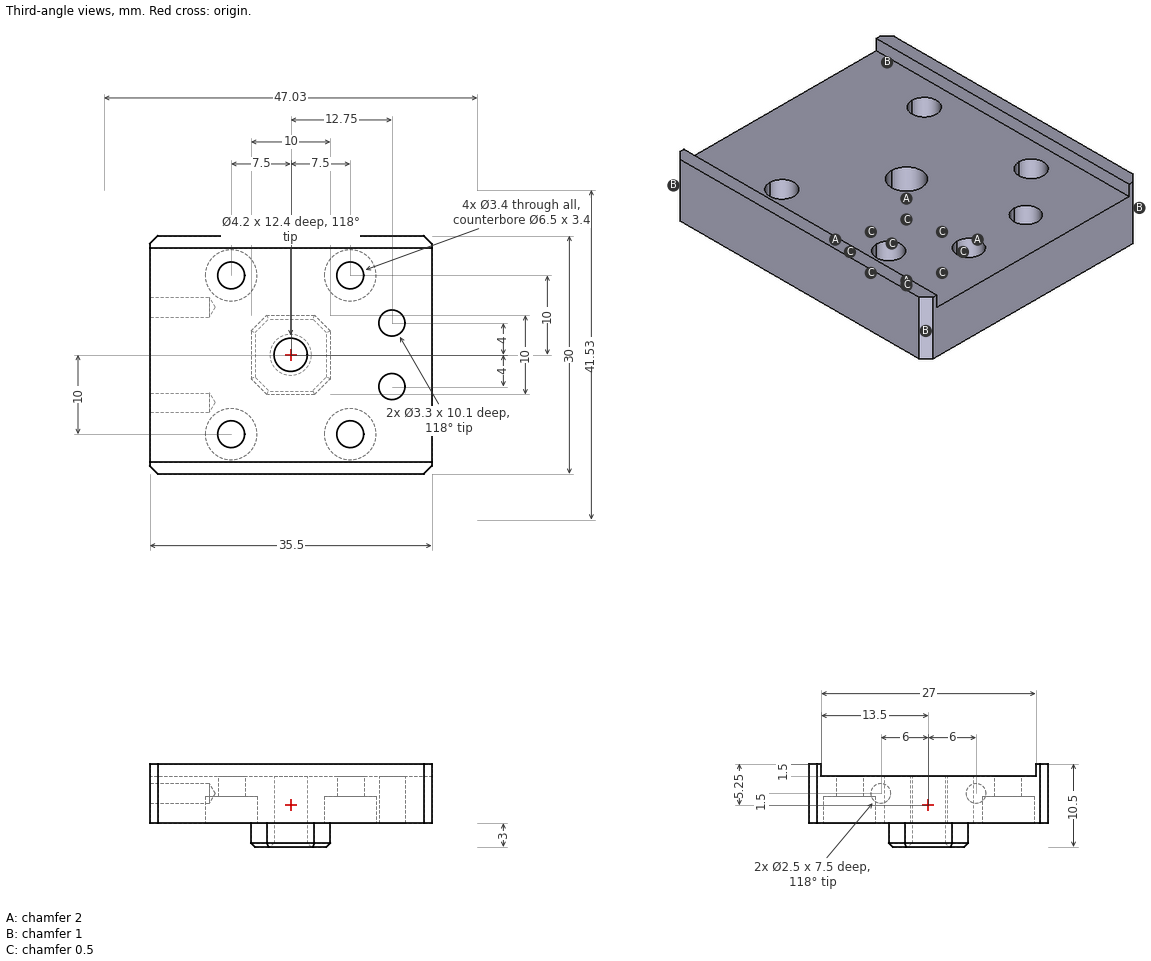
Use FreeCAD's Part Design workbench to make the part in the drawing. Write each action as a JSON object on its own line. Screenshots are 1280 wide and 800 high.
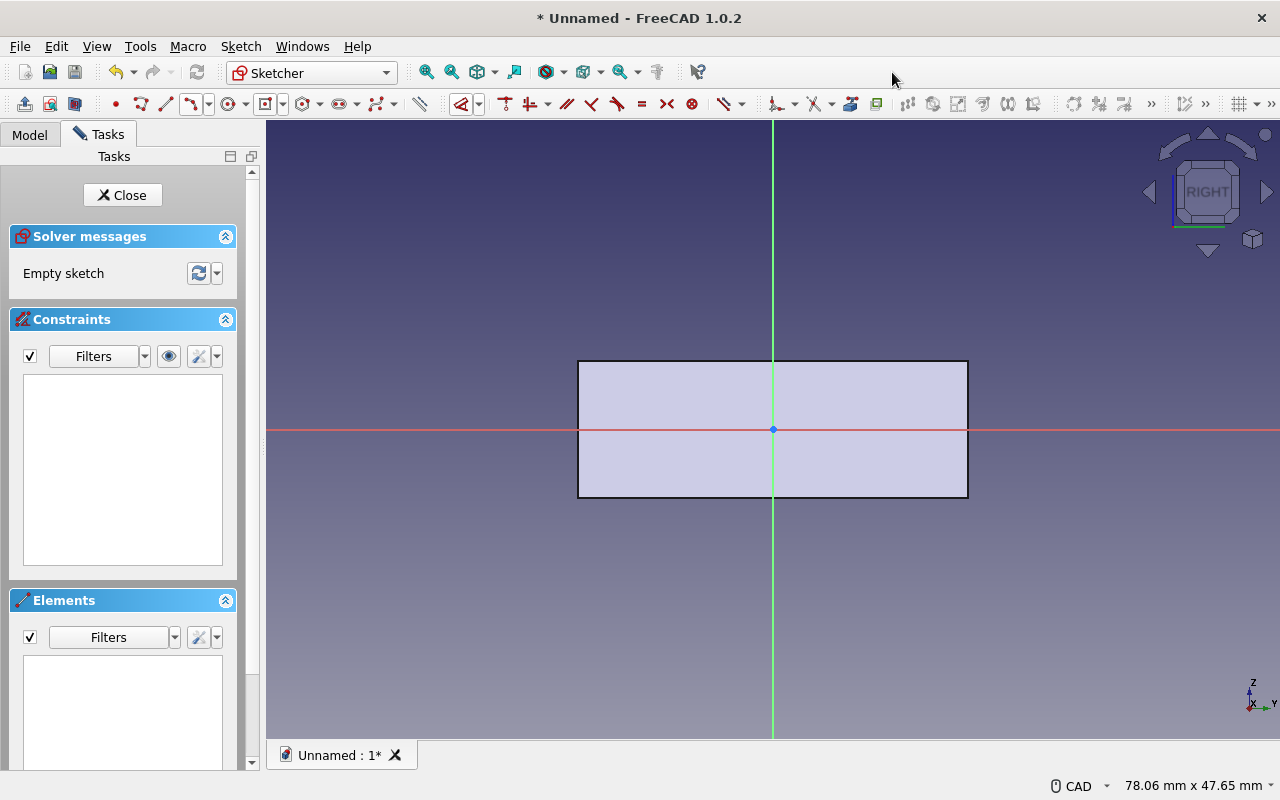
{"action": "scroll", "coordinate": [856, 354], "scroll_direction": "up", "scroll_amount": 3}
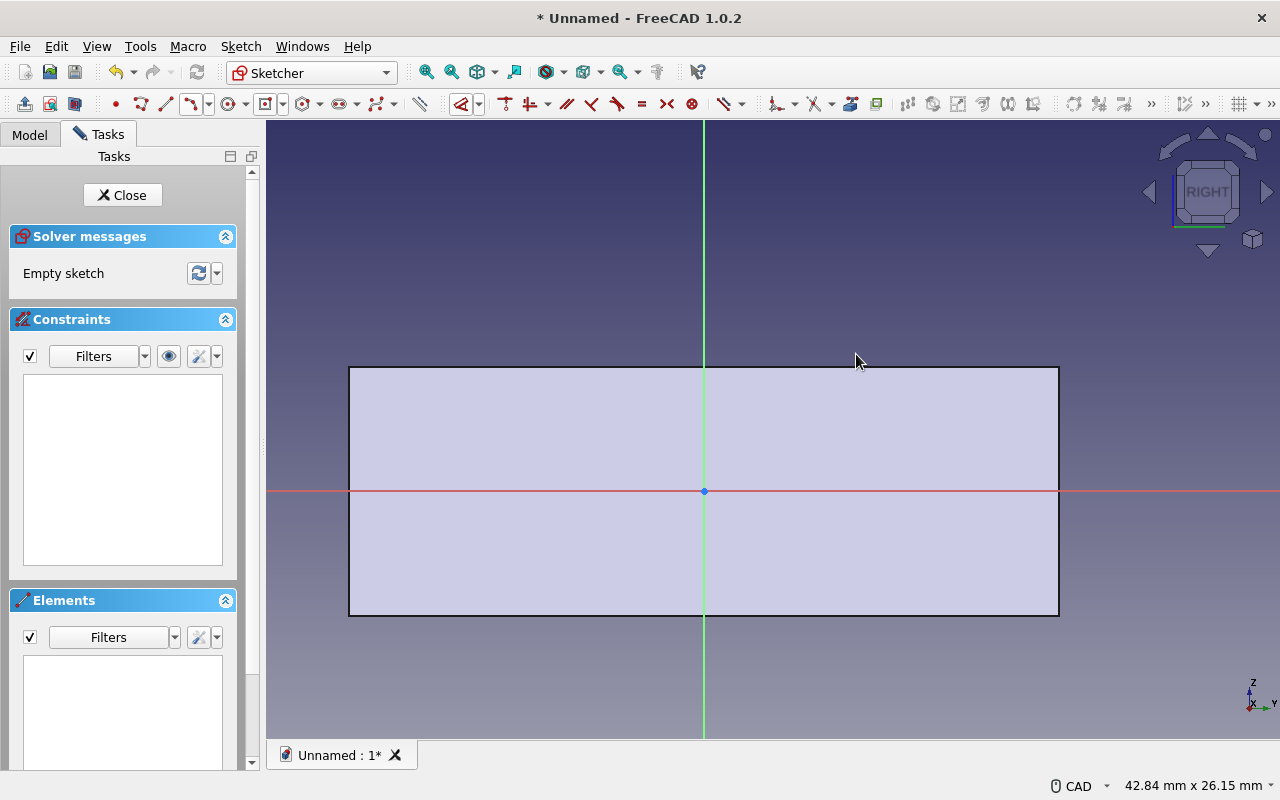
{"action": "key", "text": "g r"}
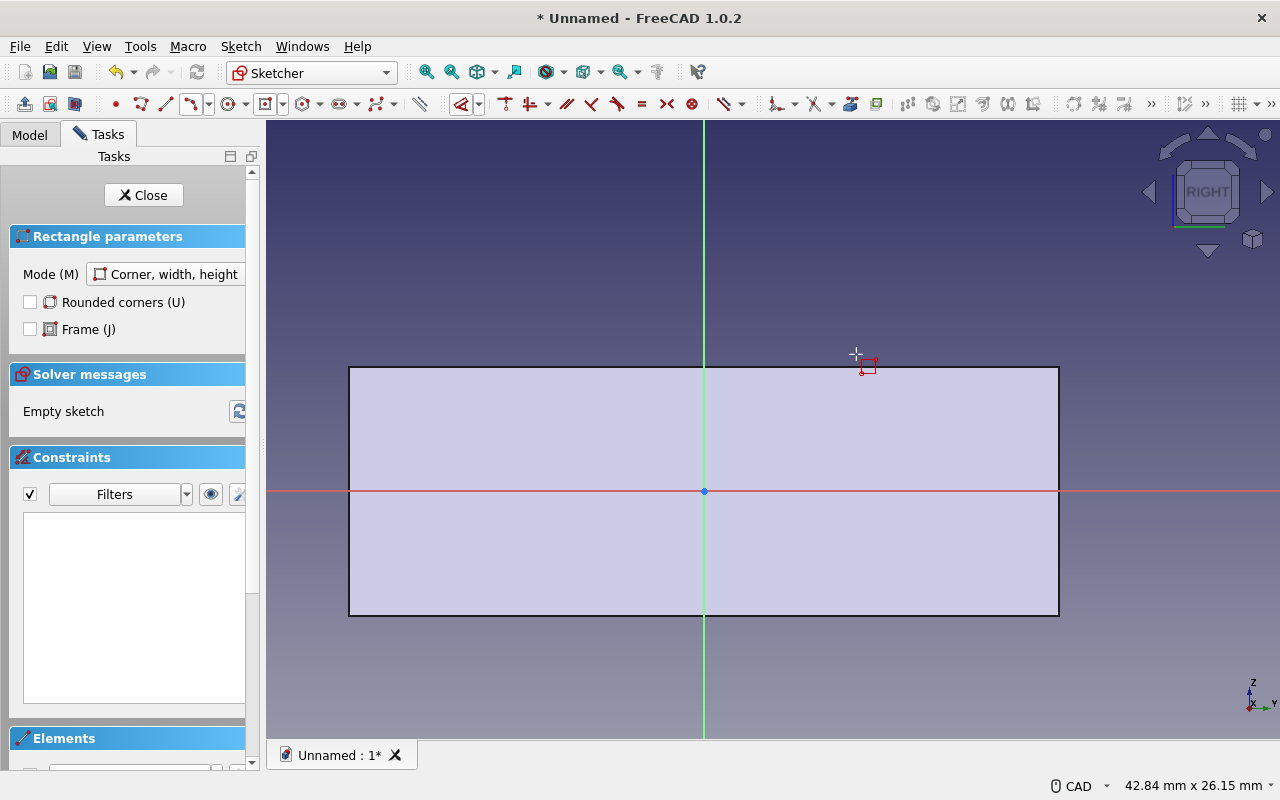
{"action": "left_click", "coordinate": [385, 367]}
{"action": "left_click", "coordinate": [1024, 402]}
{"action": "key", "text": "Escape"}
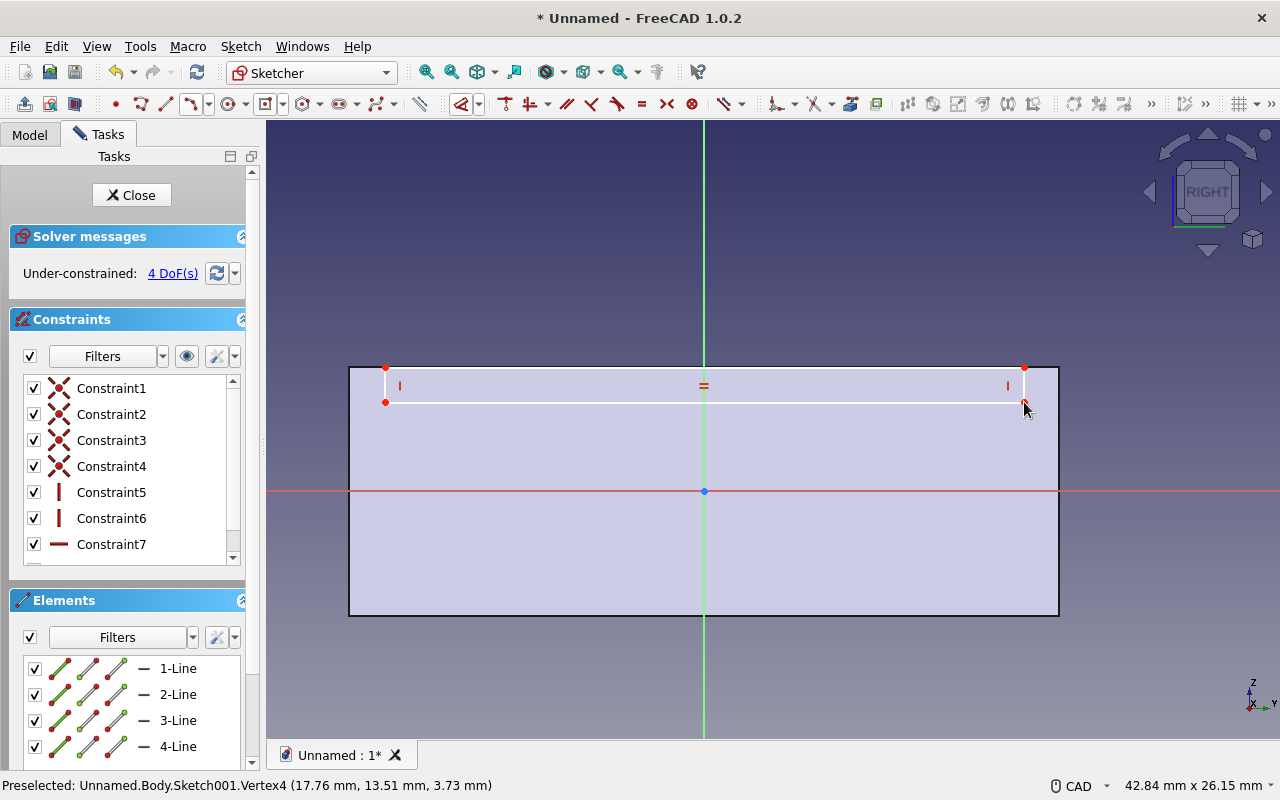
{"action": "key", "text": "d"}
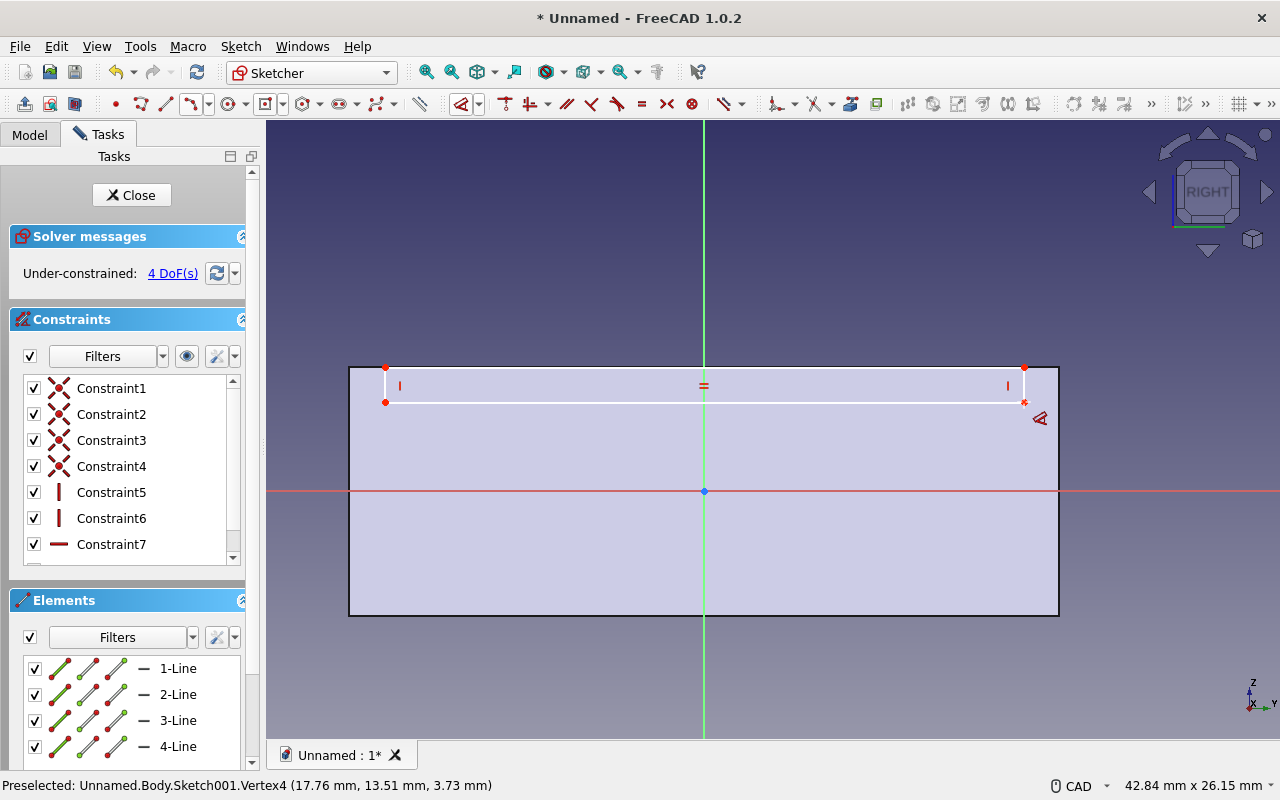
{"action": "left_click", "coordinate": [577, 403]}
{"action": "left_click", "coordinate": [558, 437]}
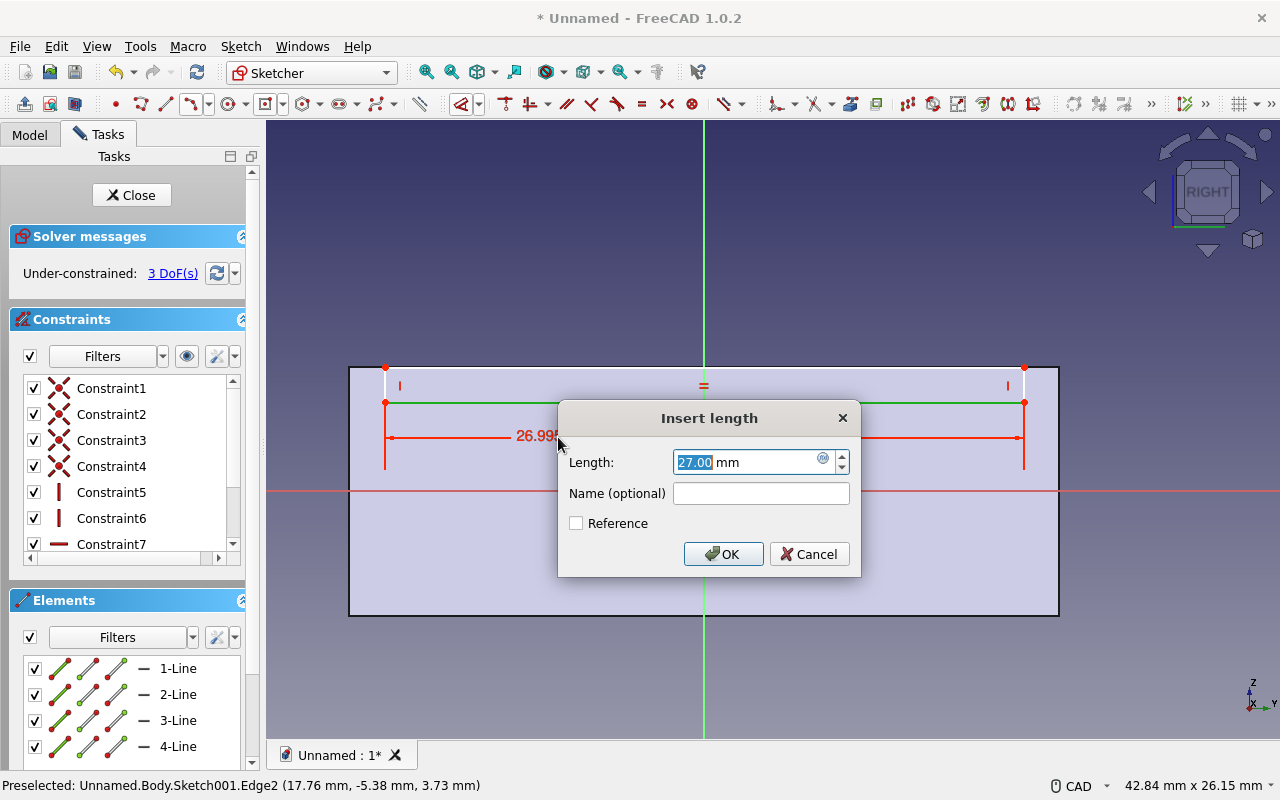
{"action": "type", "text": "27"}
{"action": "key", "text": "Return"}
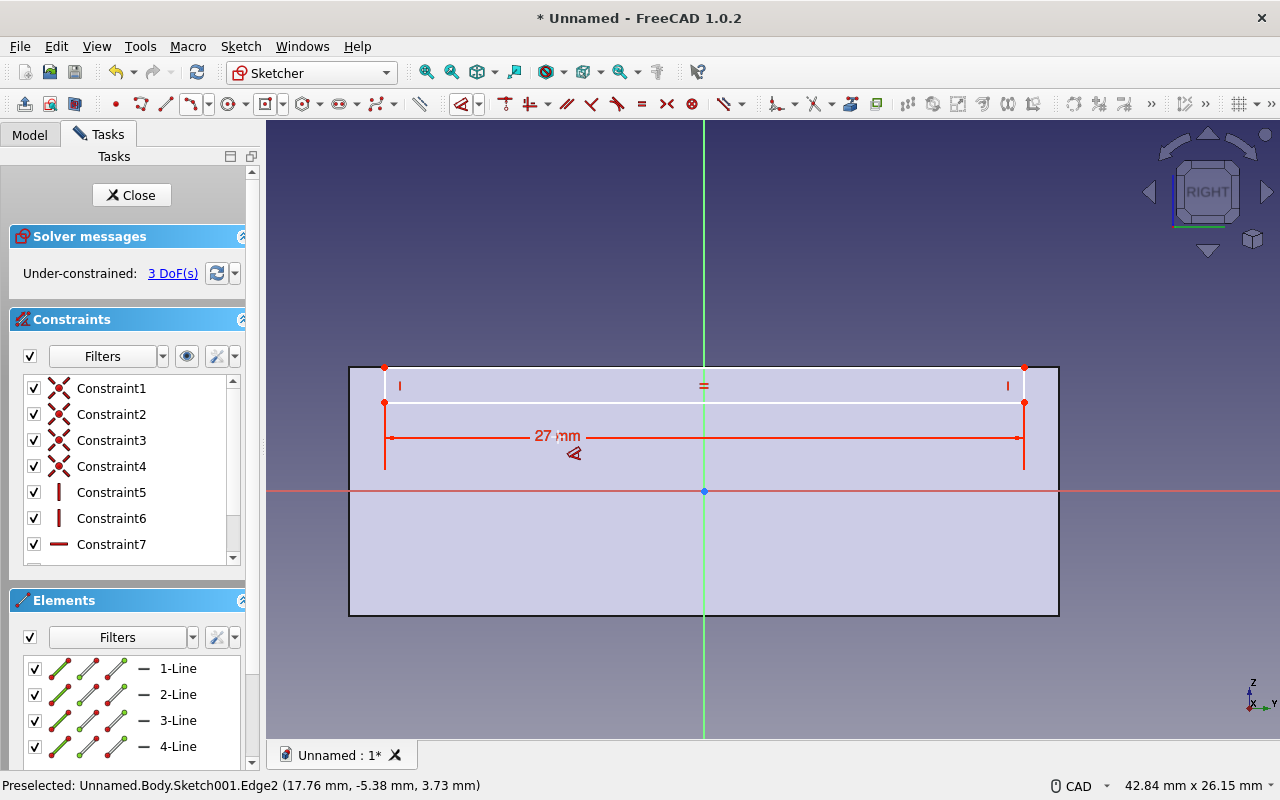
{"action": "scroll", "coordinate": [385, 379], "scroll_direction": "up", "scroll_amount": 2}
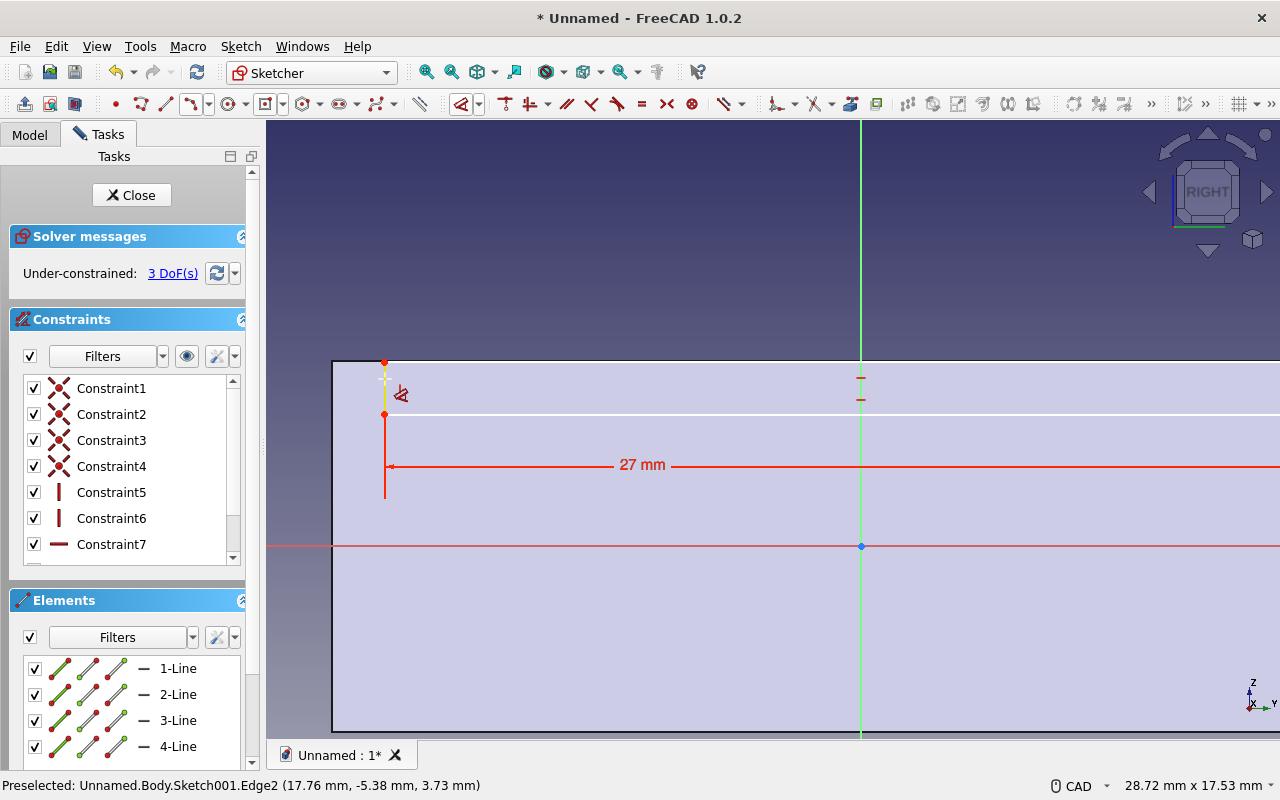
{"action": "left_click", "coordinate": [385, 378]}
{"action": "left_click", "coordinate": [351, 388]}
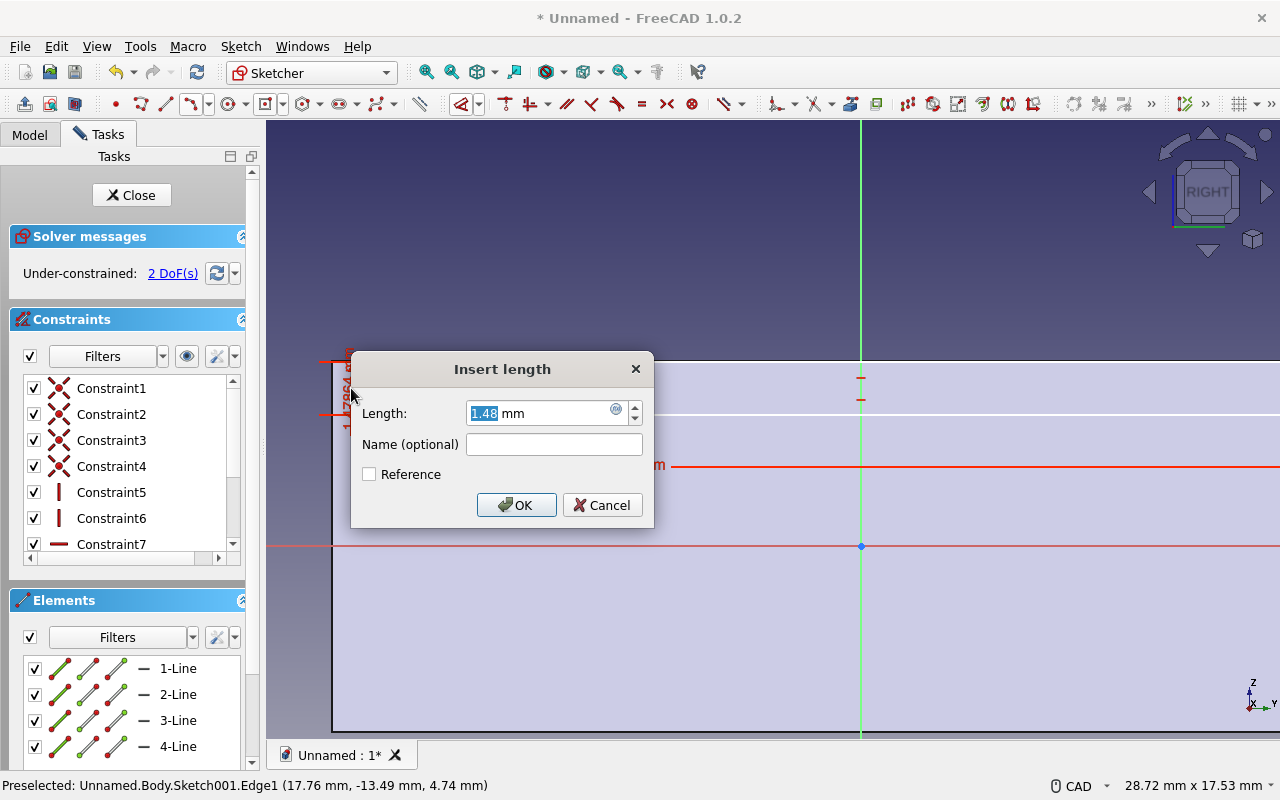
{"action": "type", "text": "1.5"}
{"action": "key", "text": "Return"}